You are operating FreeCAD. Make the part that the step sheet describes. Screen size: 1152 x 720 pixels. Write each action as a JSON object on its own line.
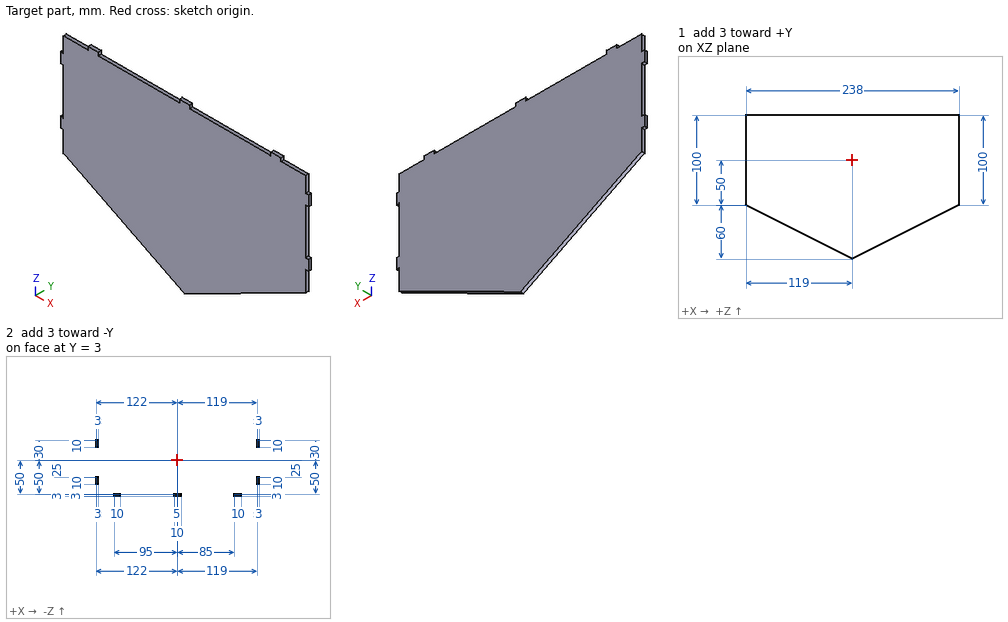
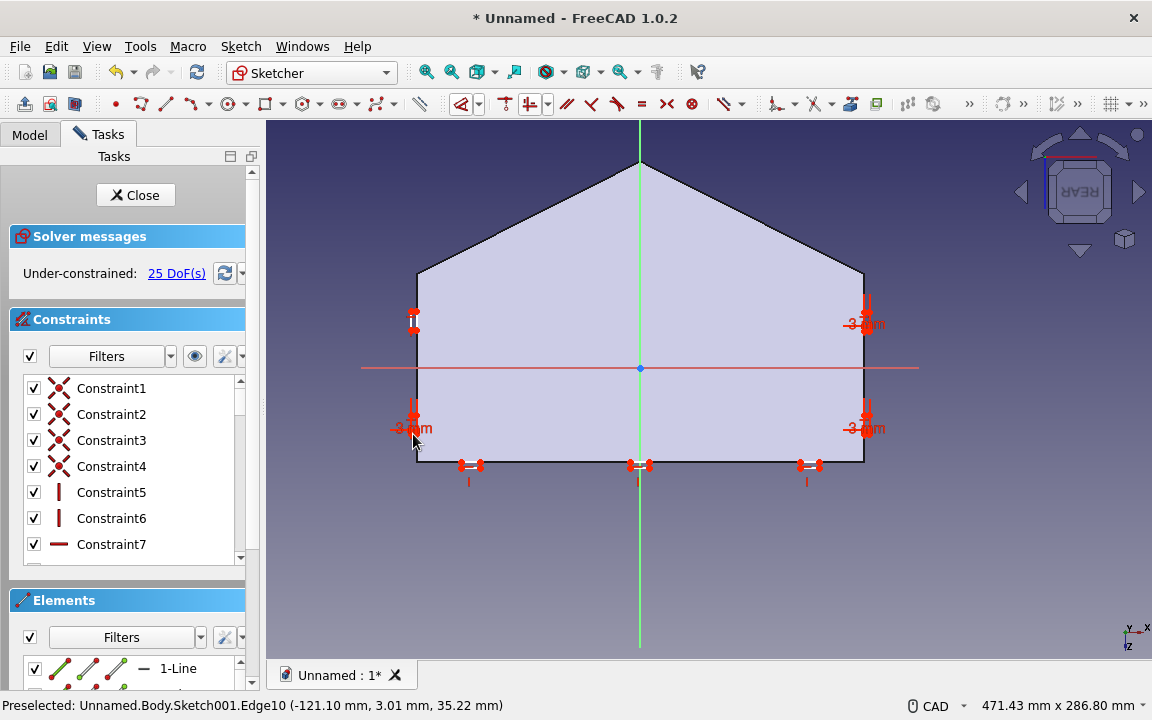
{"action": "scroll", "coordinate": [413, 331], "scroll_direction": "up", "scroll_amount": 11}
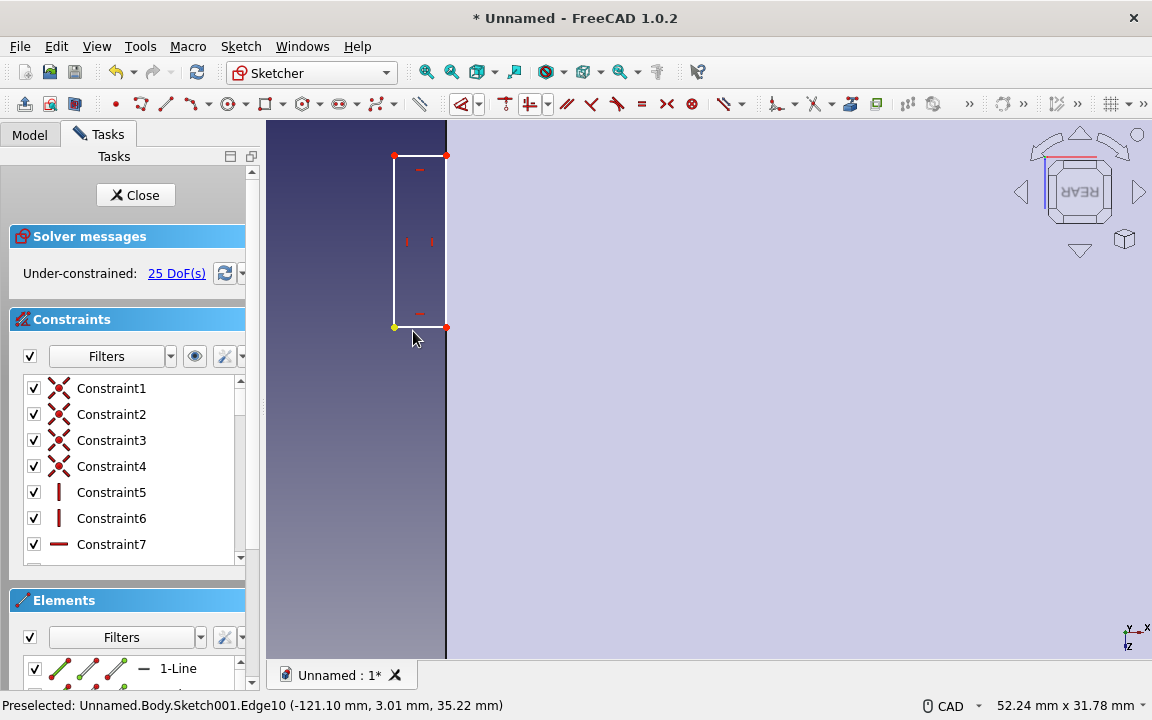
{"action": "left_click", "coordinate": [410, 327]}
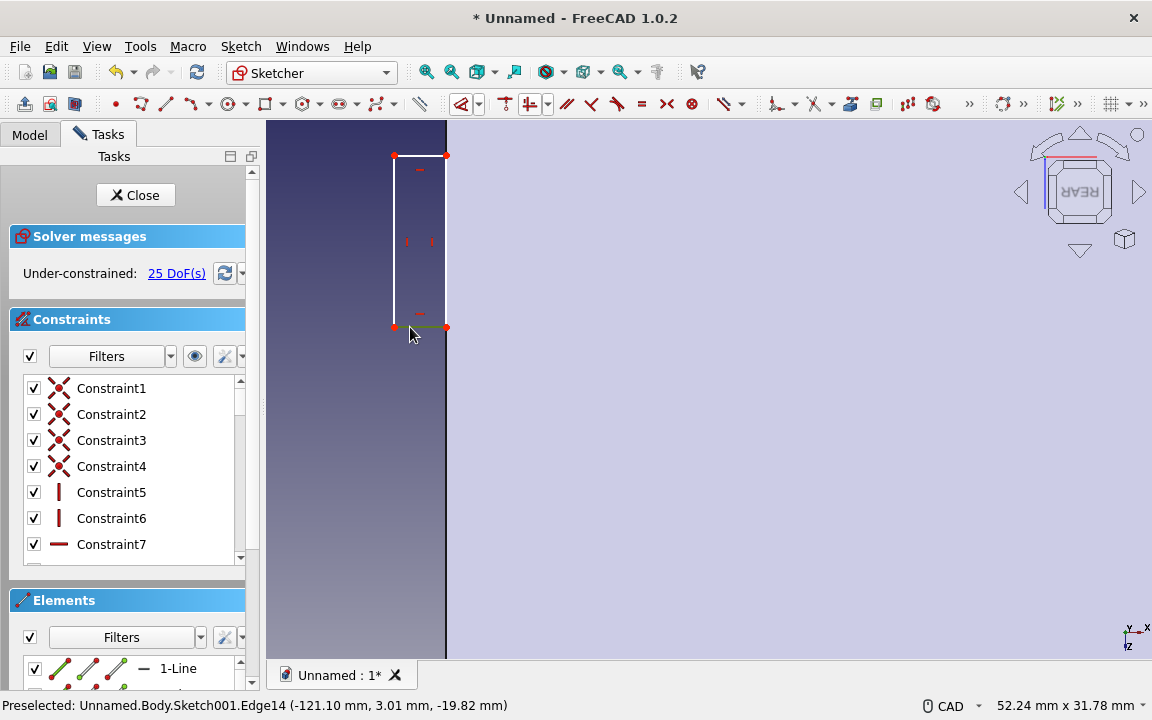
{"action": "left_click", "coordinate": [478, 104]}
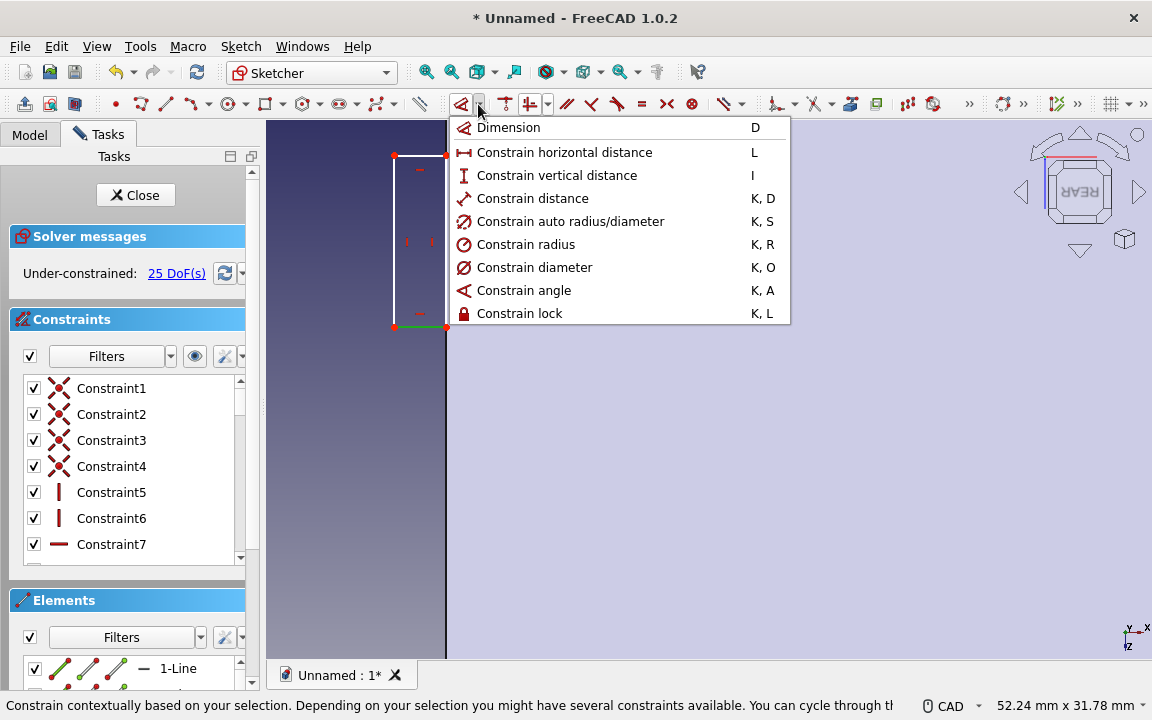
{"action": "left_click", "coordinate": [620, 152]}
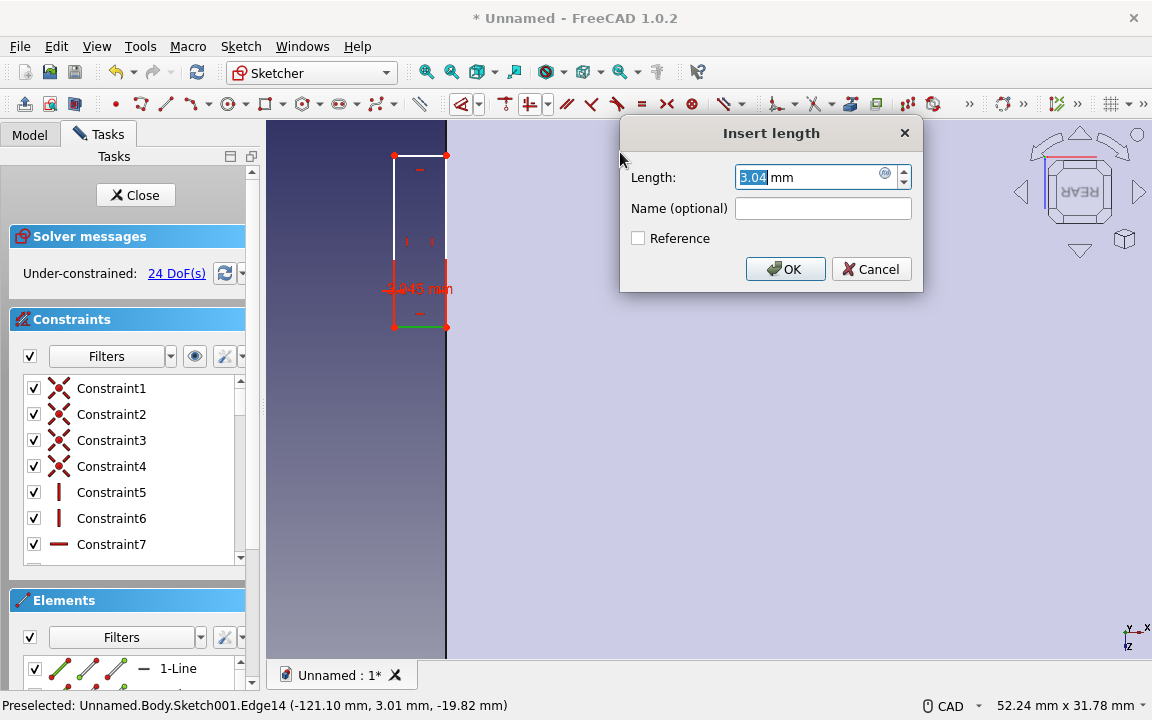
{"action": "type", "text": "3"}
{"action": "key", "text": "Return"}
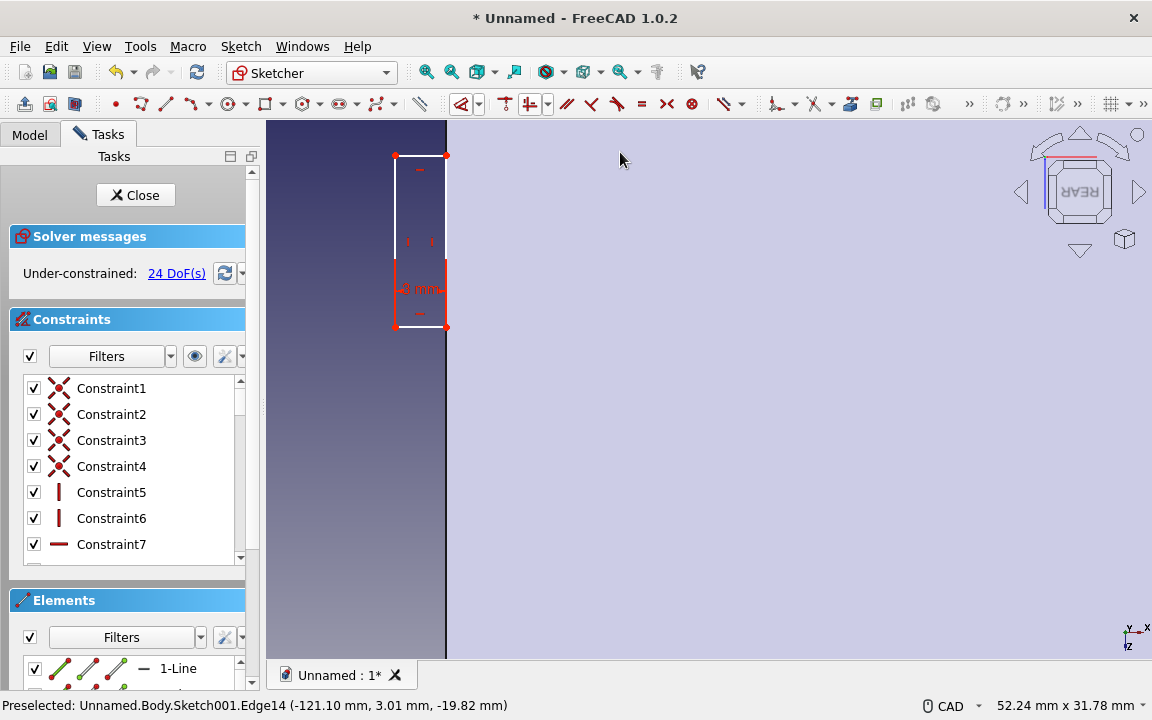
{"action": "scroll", "coordinate": [413, 331], "scroll_direction": "down", "scroll_amount": 11}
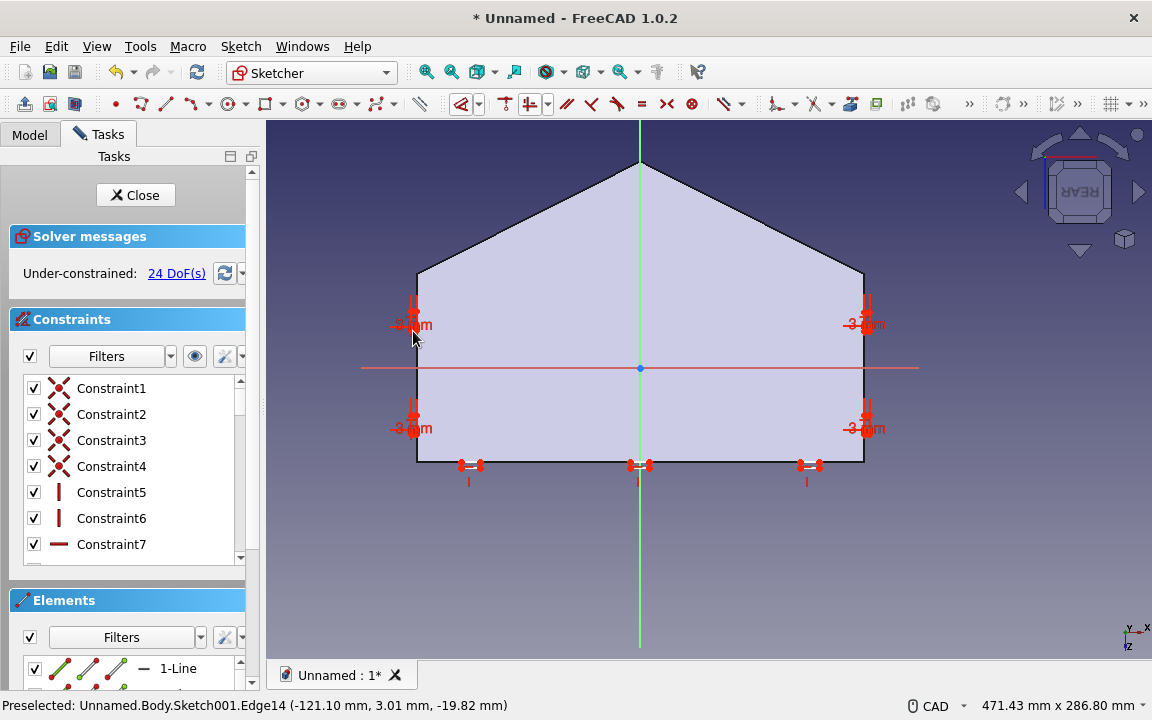
{"action": "scroll", "coordinate": [462, 464], "scroll_direction": "up", "scroll_amount": 11}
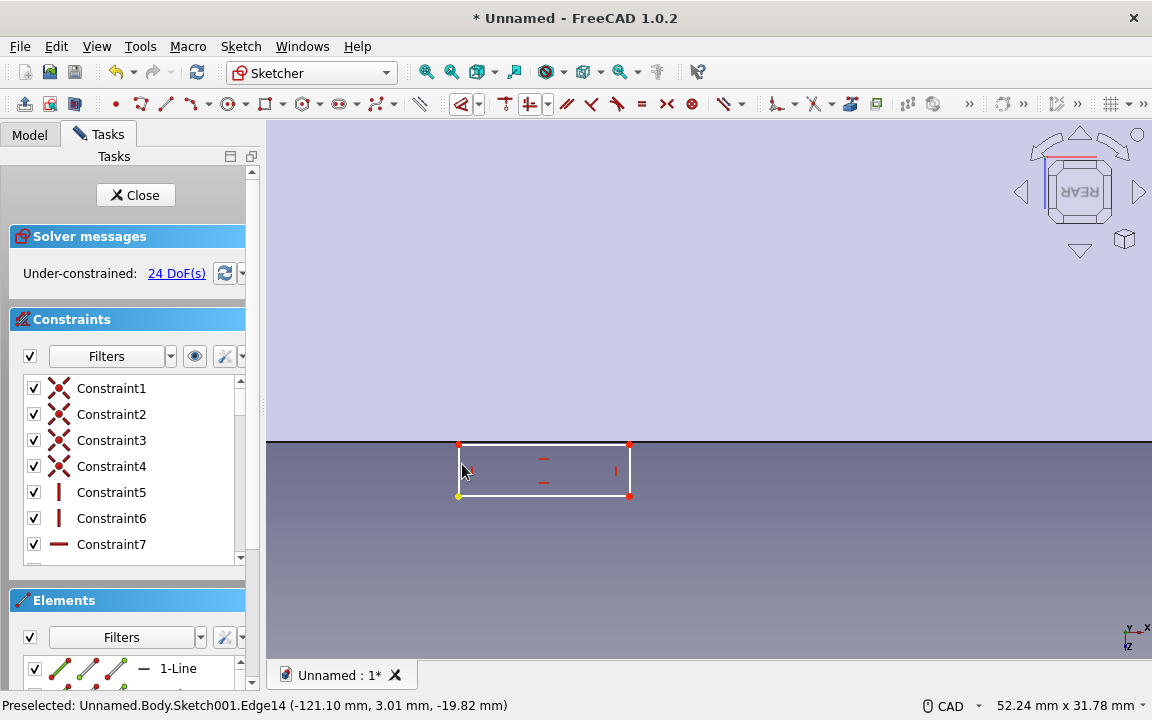
{"action": "left_click", "coordinate": [459, 460]}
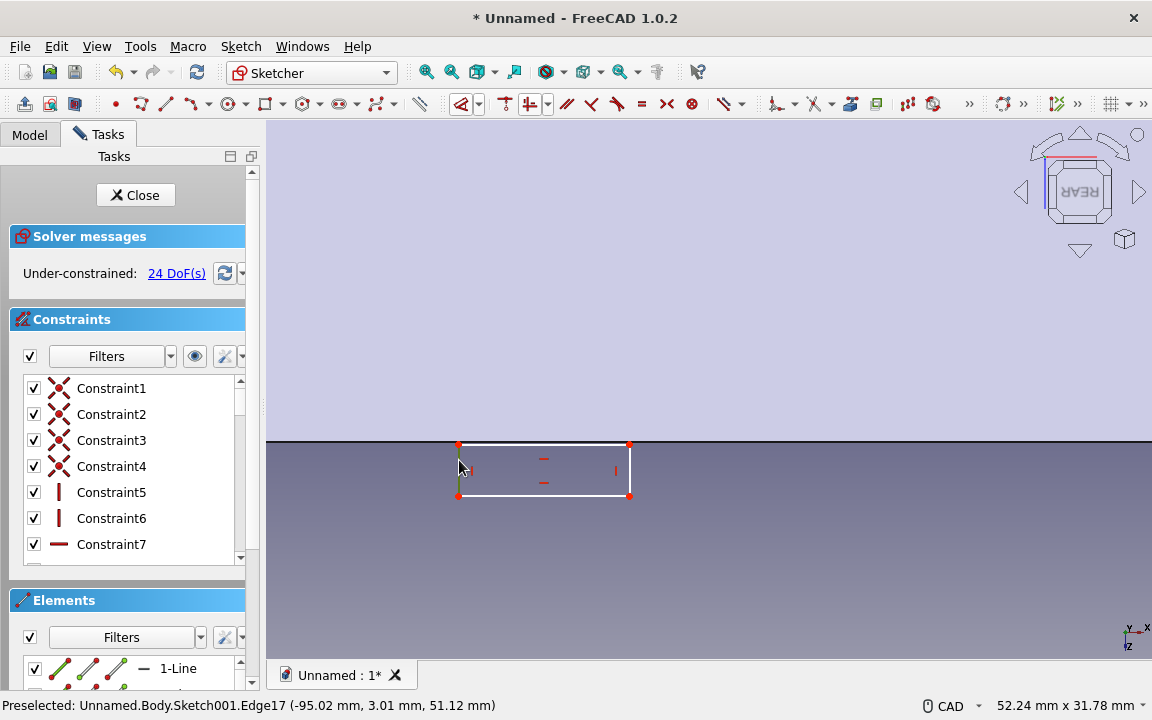
{"action": "key", "text": "i"}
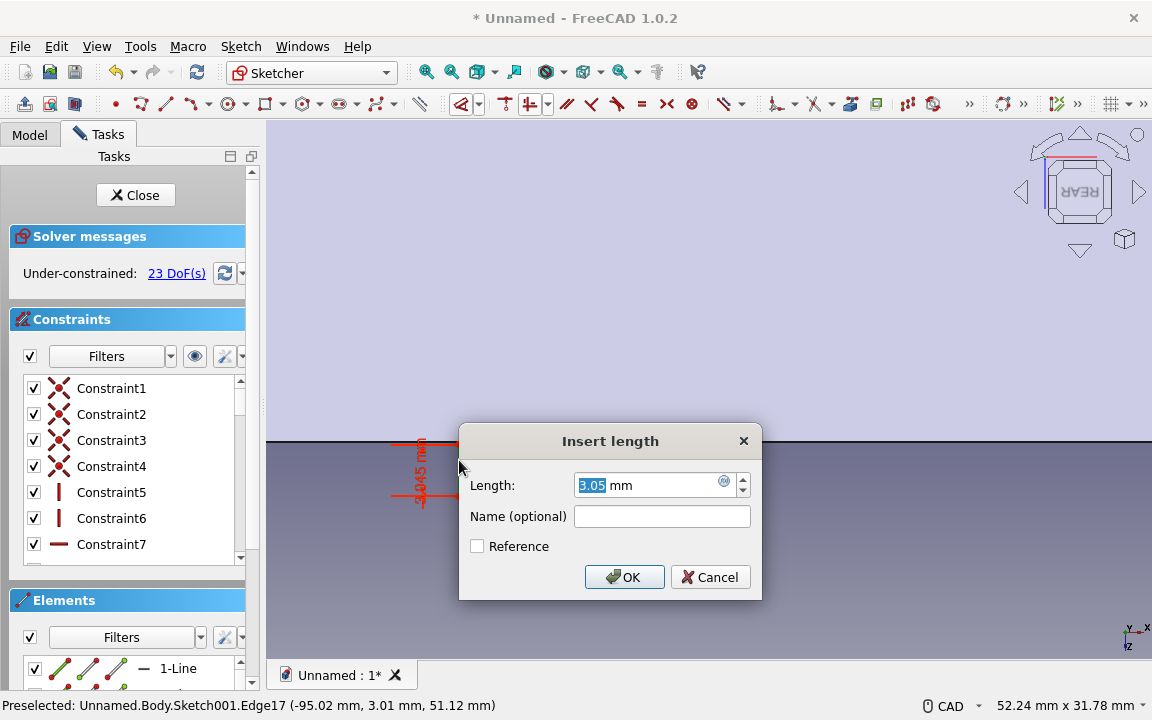
{"action": "type", "text": "3"}
{"action": "key", "text": "Return"}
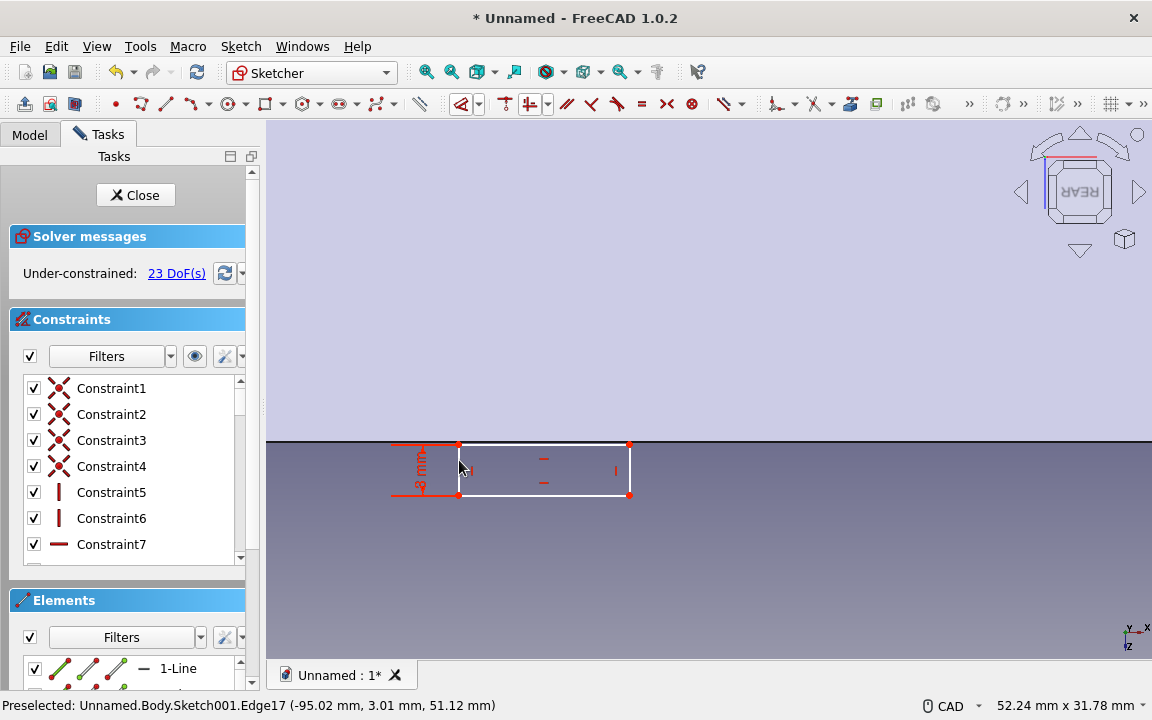
{"action": "scroll", "coordinate": [462, 464], "scroll_direction": "down", "scroll_amount": 11}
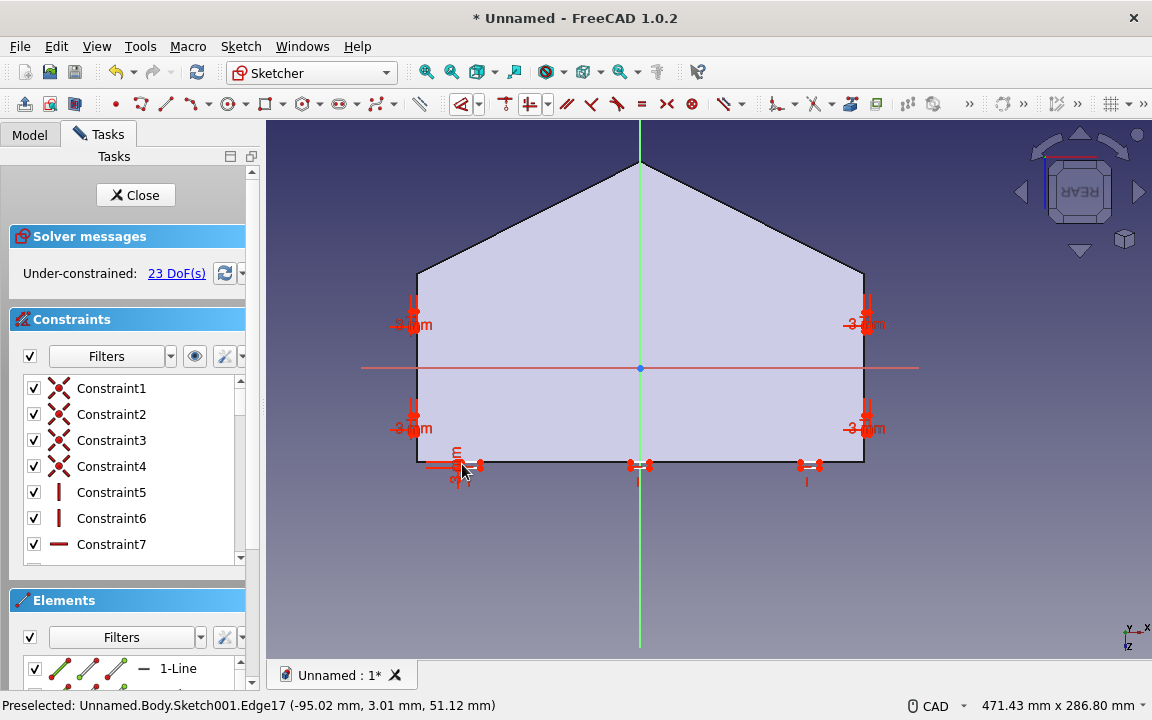
{"action": "scroll", "coordinate": [800, 464], "scroll_direction": "up", "scroll_amount": 11}